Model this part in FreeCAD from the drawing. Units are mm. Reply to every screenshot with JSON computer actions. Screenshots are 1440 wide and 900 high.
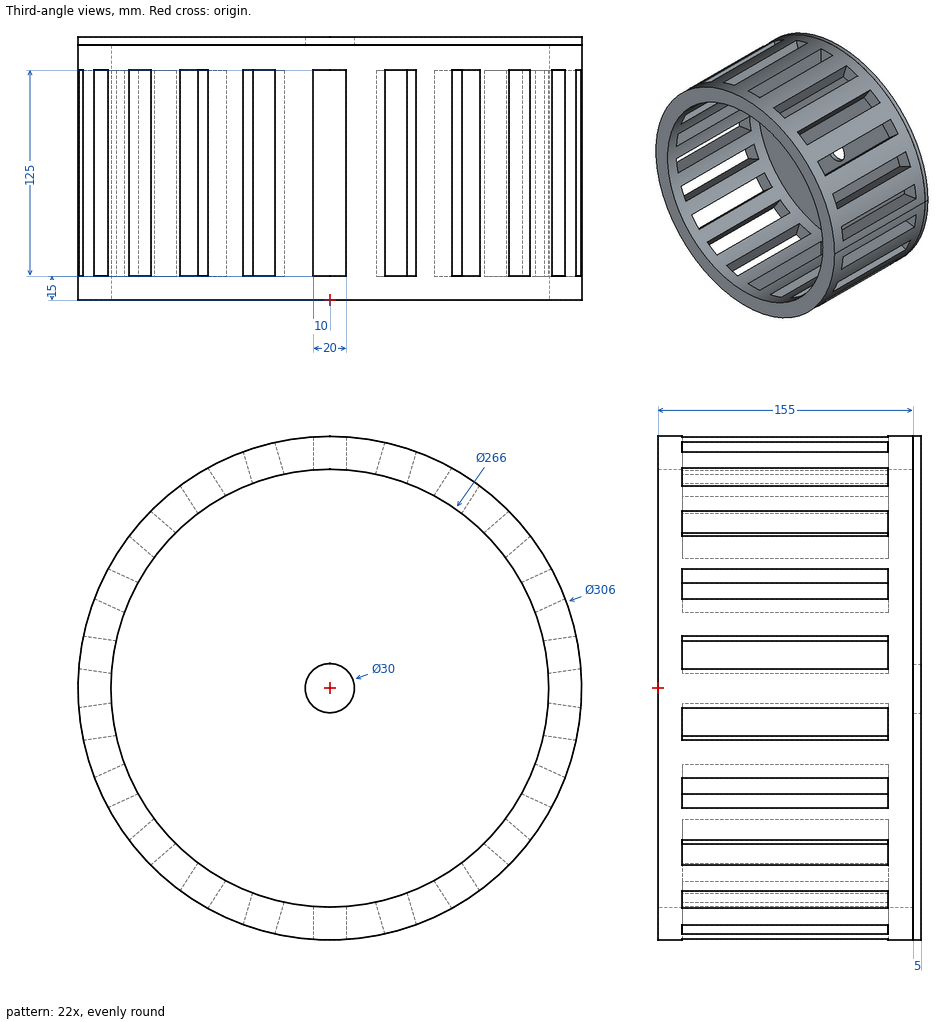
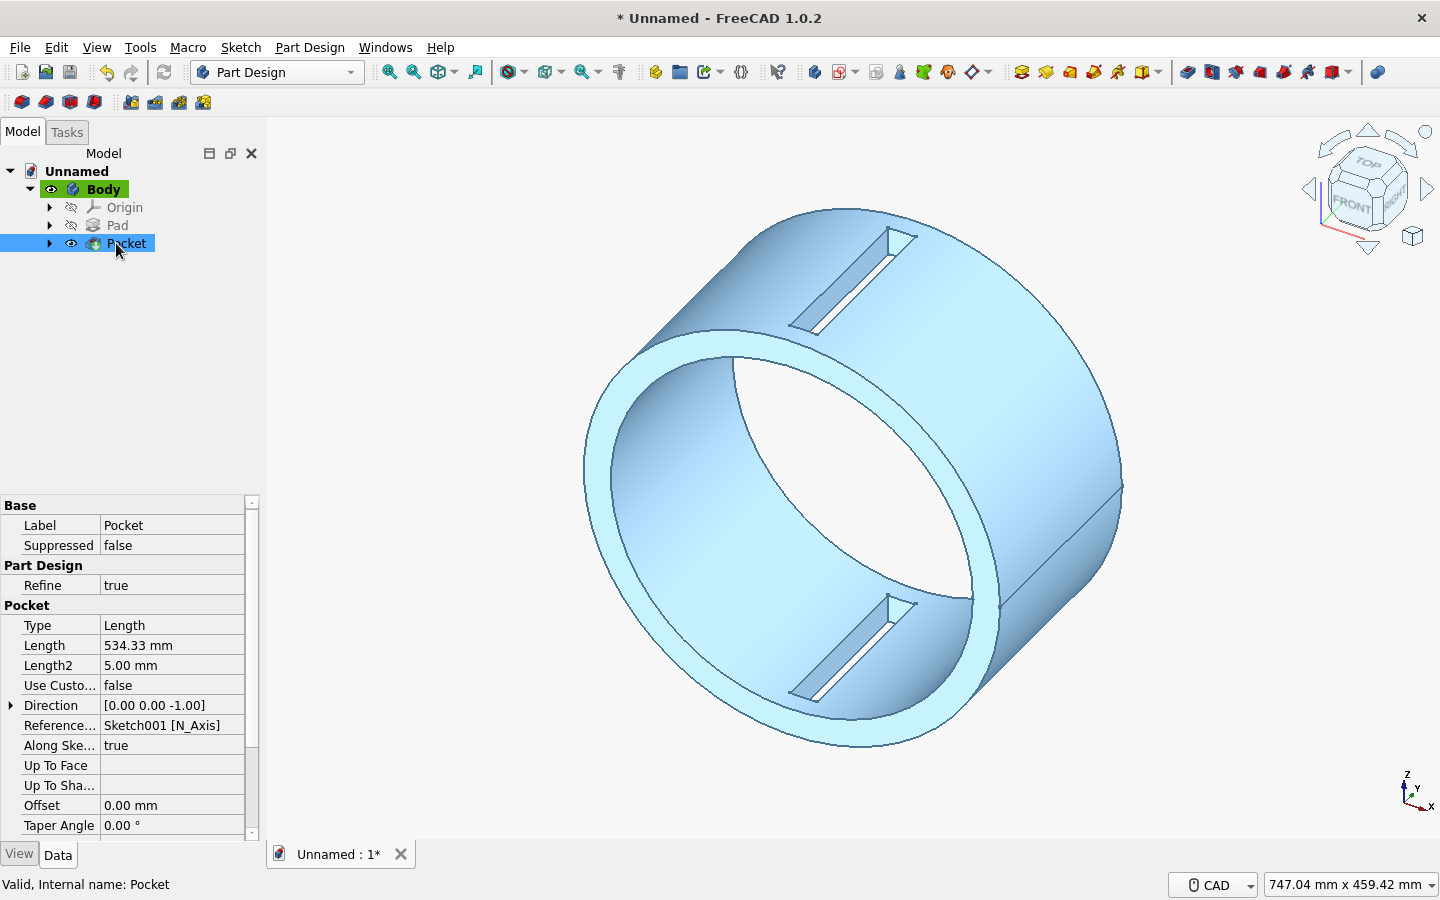
{"action": "left_click", "coordinate": [180, 102]}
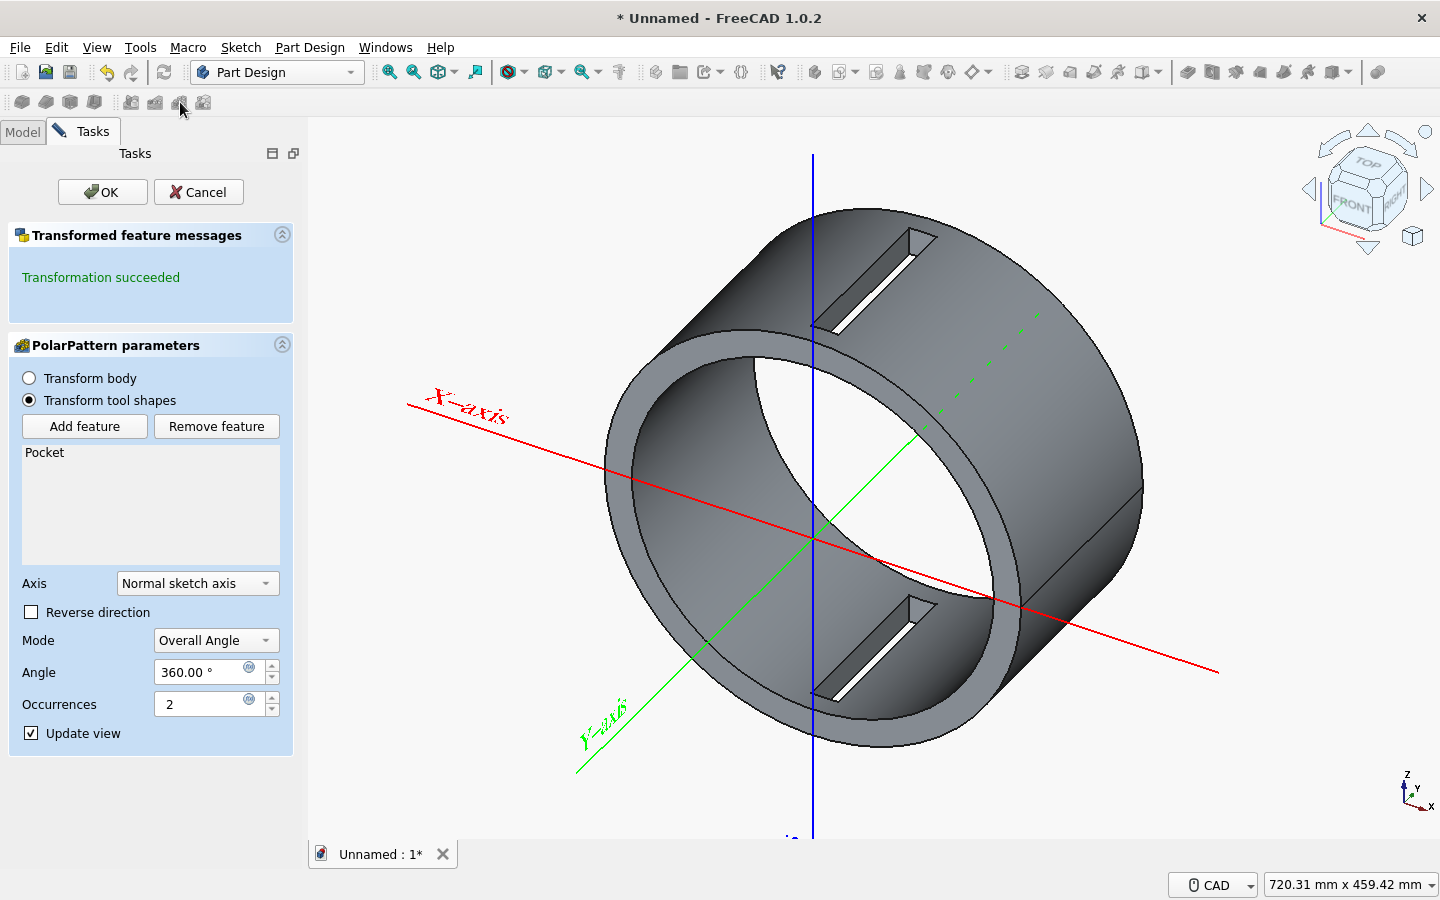
{"action": "left_click", "coordinate": [198, 584]}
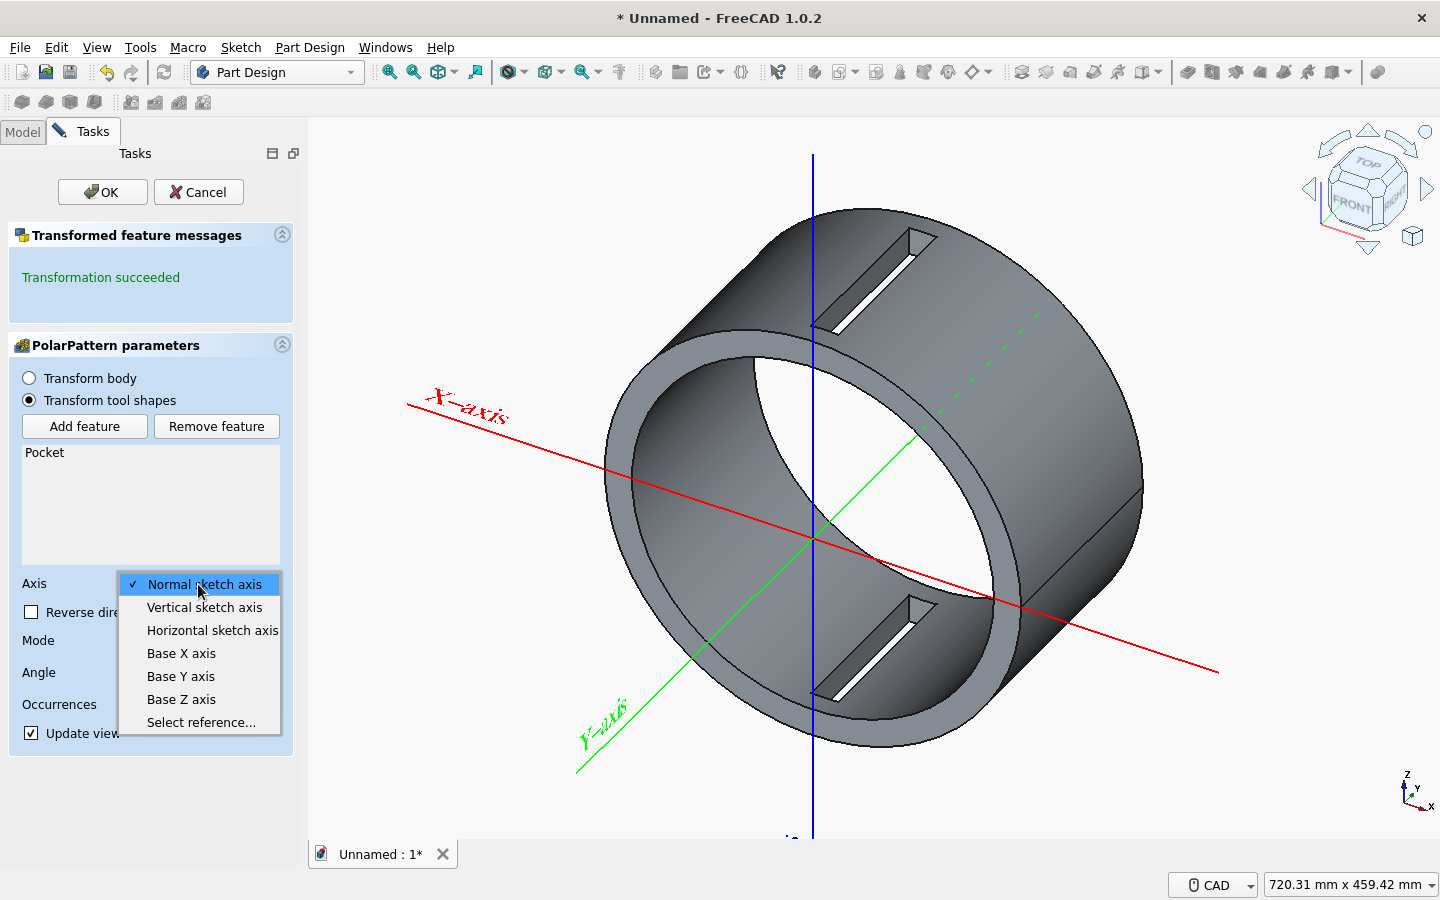
{"action": "left_click", "coordinate": [198, 676]}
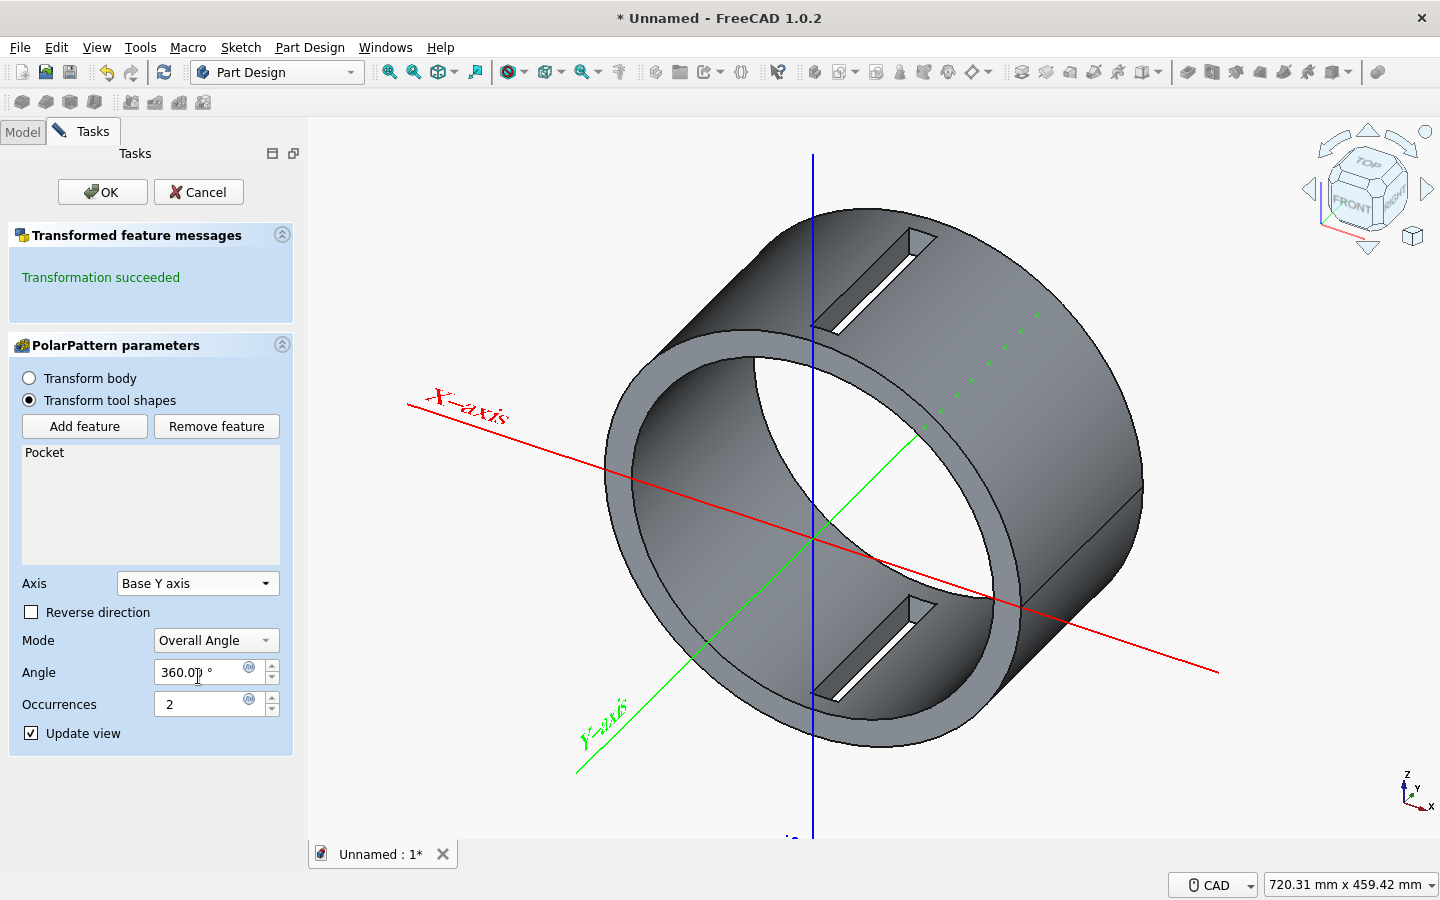
{"action": "triple_click", "coordinate": [209, 704]}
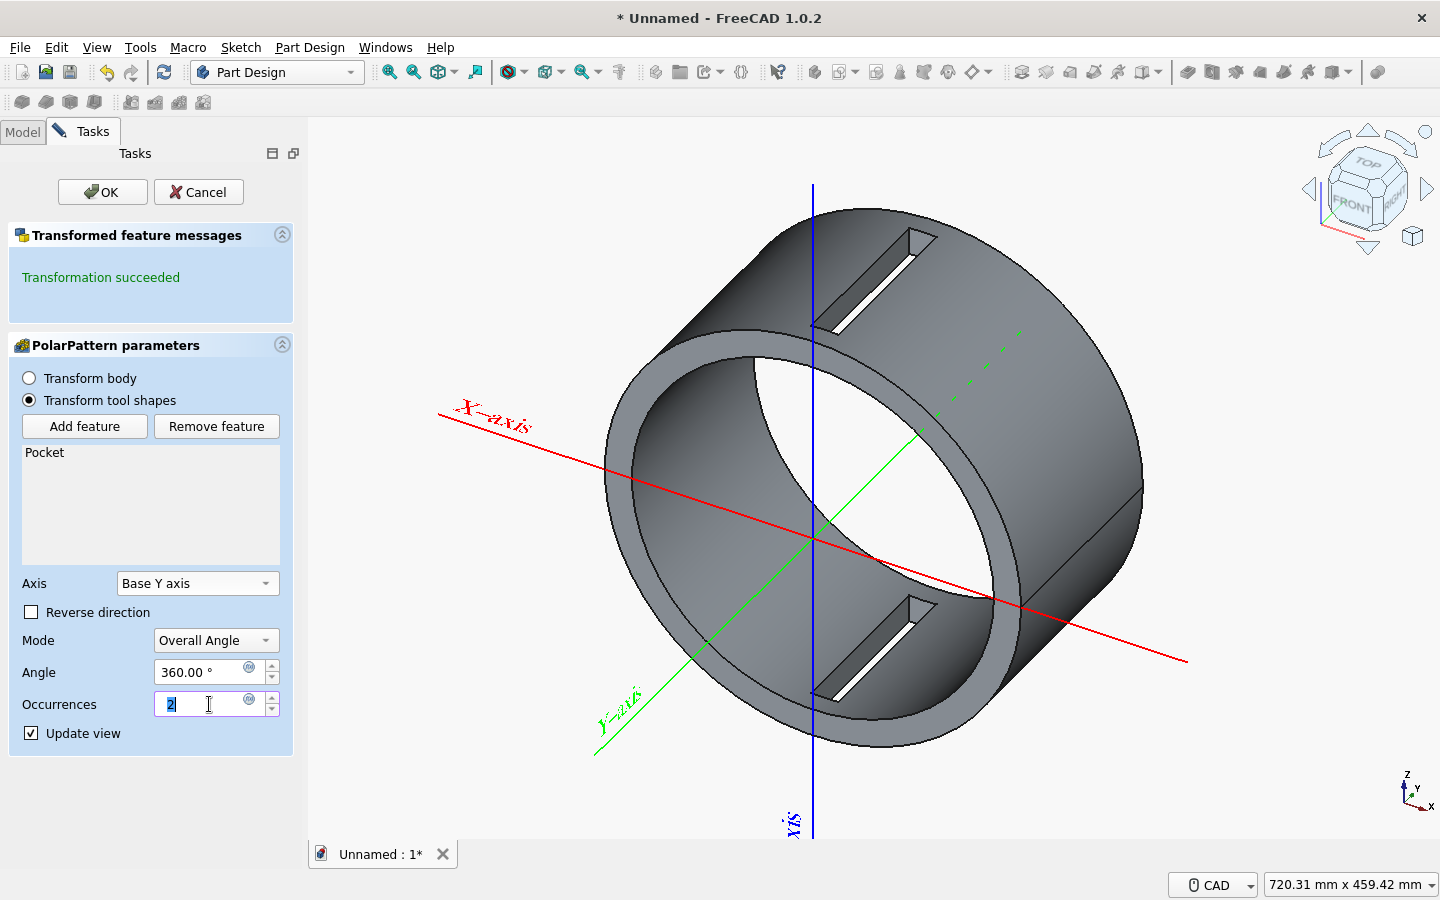
{"action": "type", "text": "22"}
{"action": "key", "text": "Tab"}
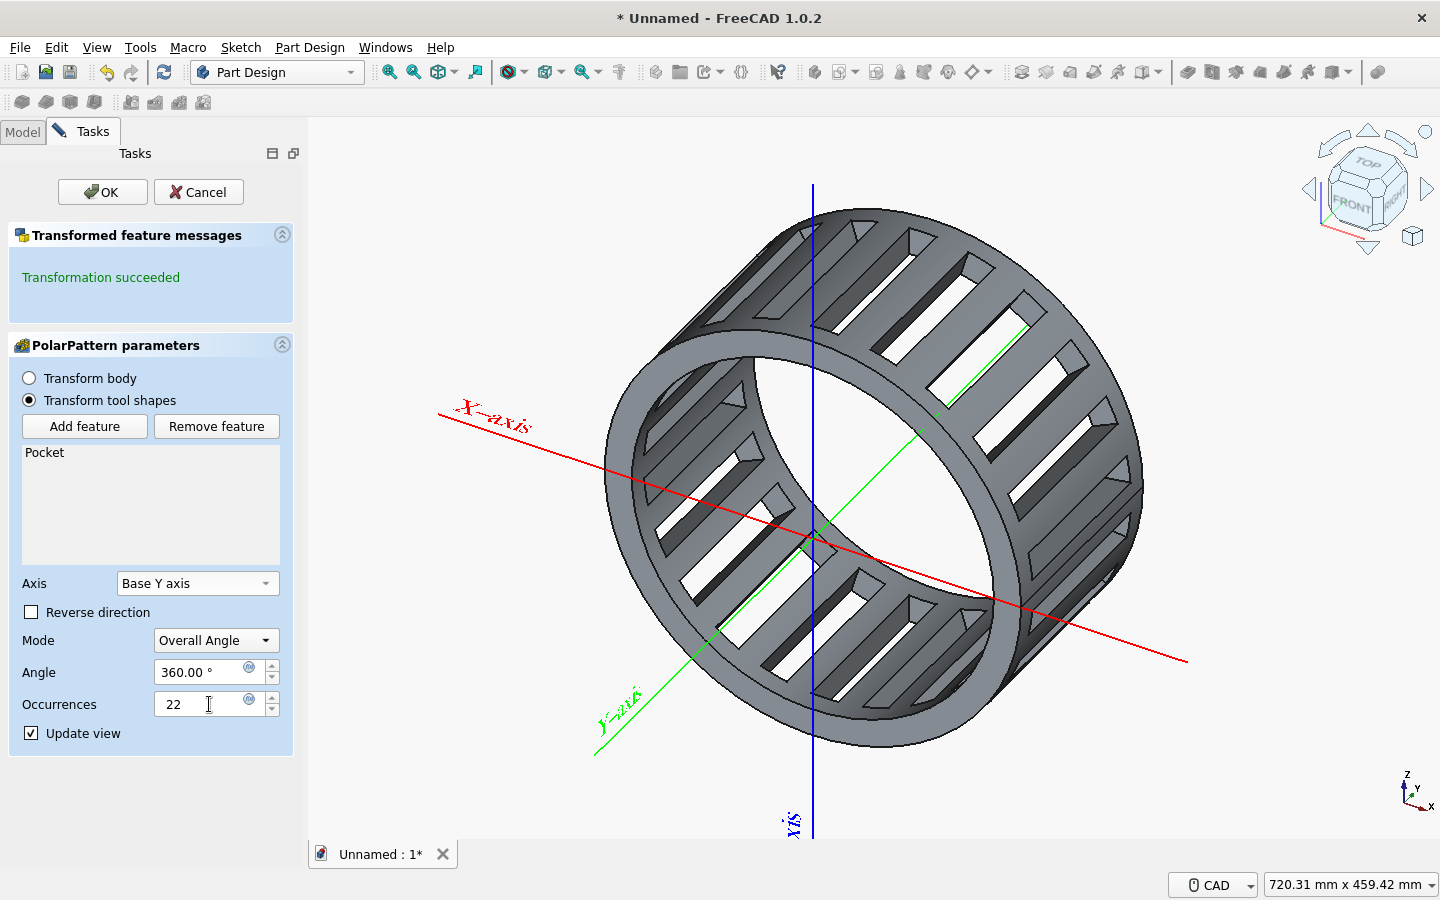
{"action": "left_click", "coordinate": [103, 192]}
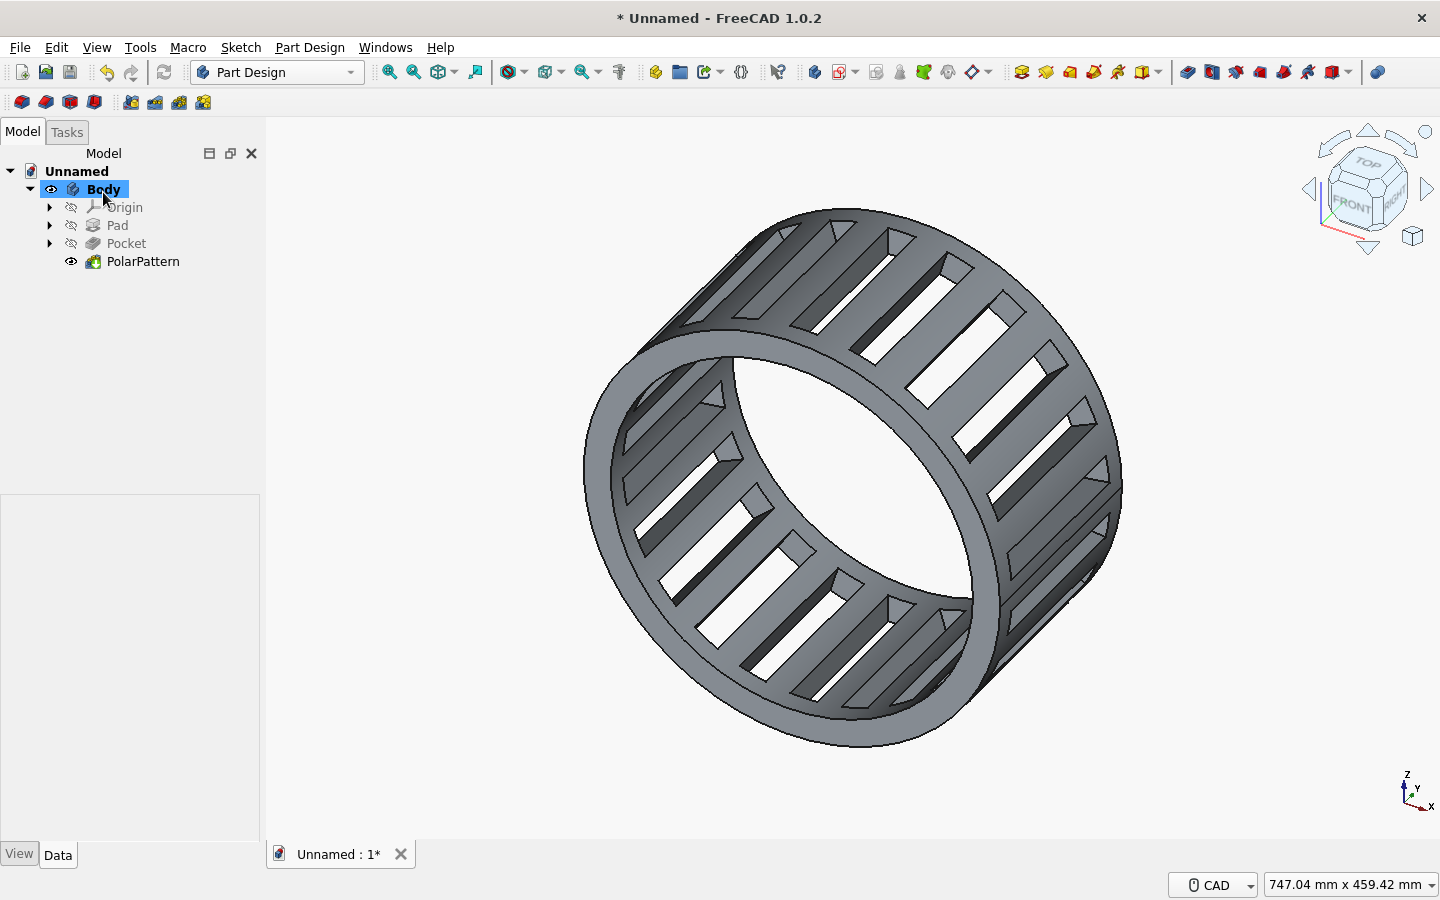
{"action": "left_click", "coordinate": [816, 72]}